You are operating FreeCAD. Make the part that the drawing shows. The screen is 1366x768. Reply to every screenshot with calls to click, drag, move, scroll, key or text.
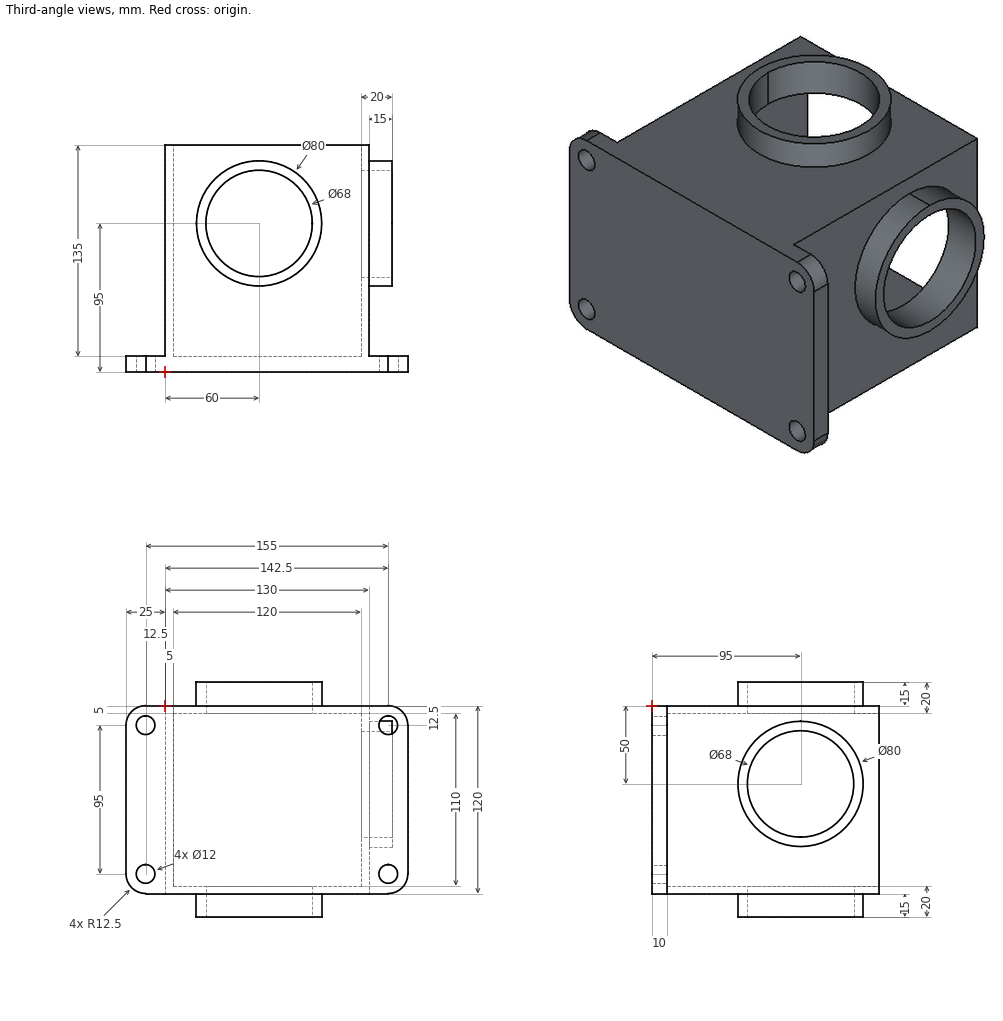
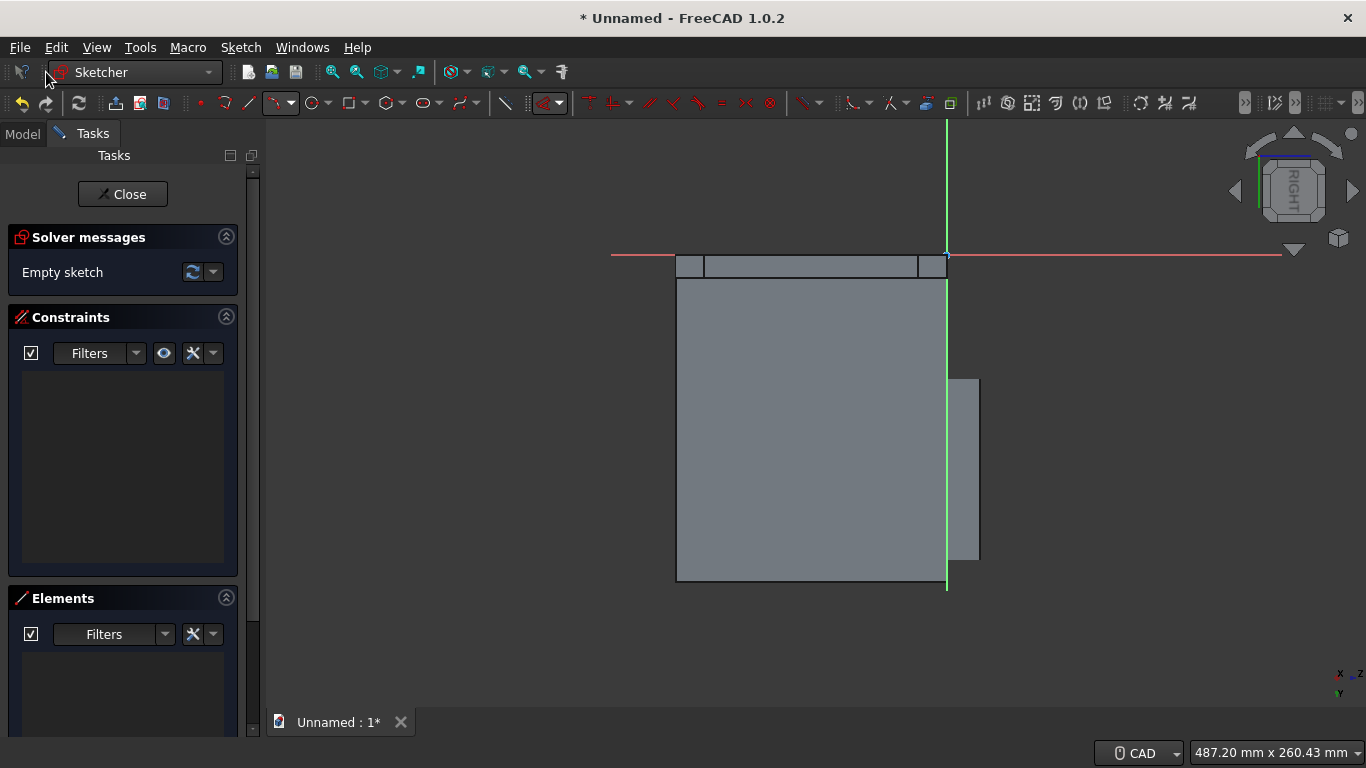
click(312, 104)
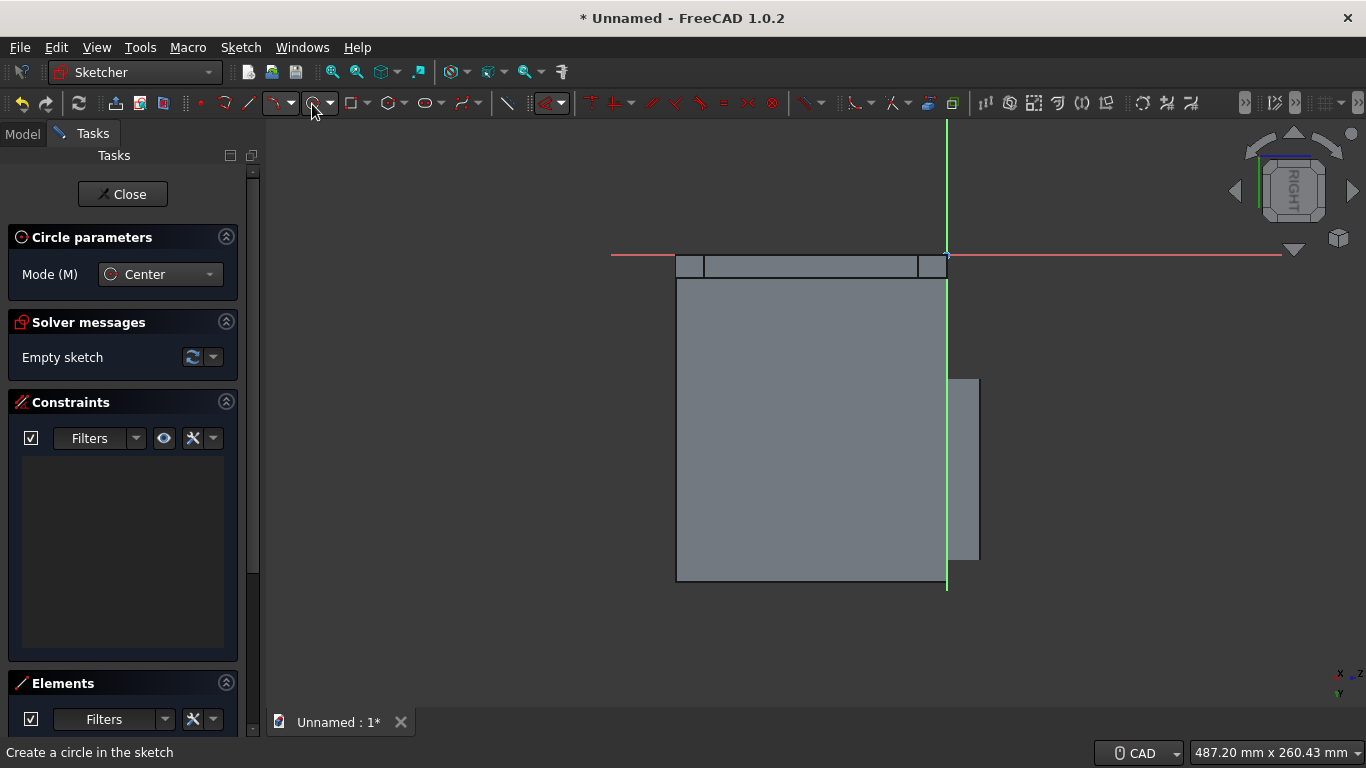
click(834, 470)
move(898, 406)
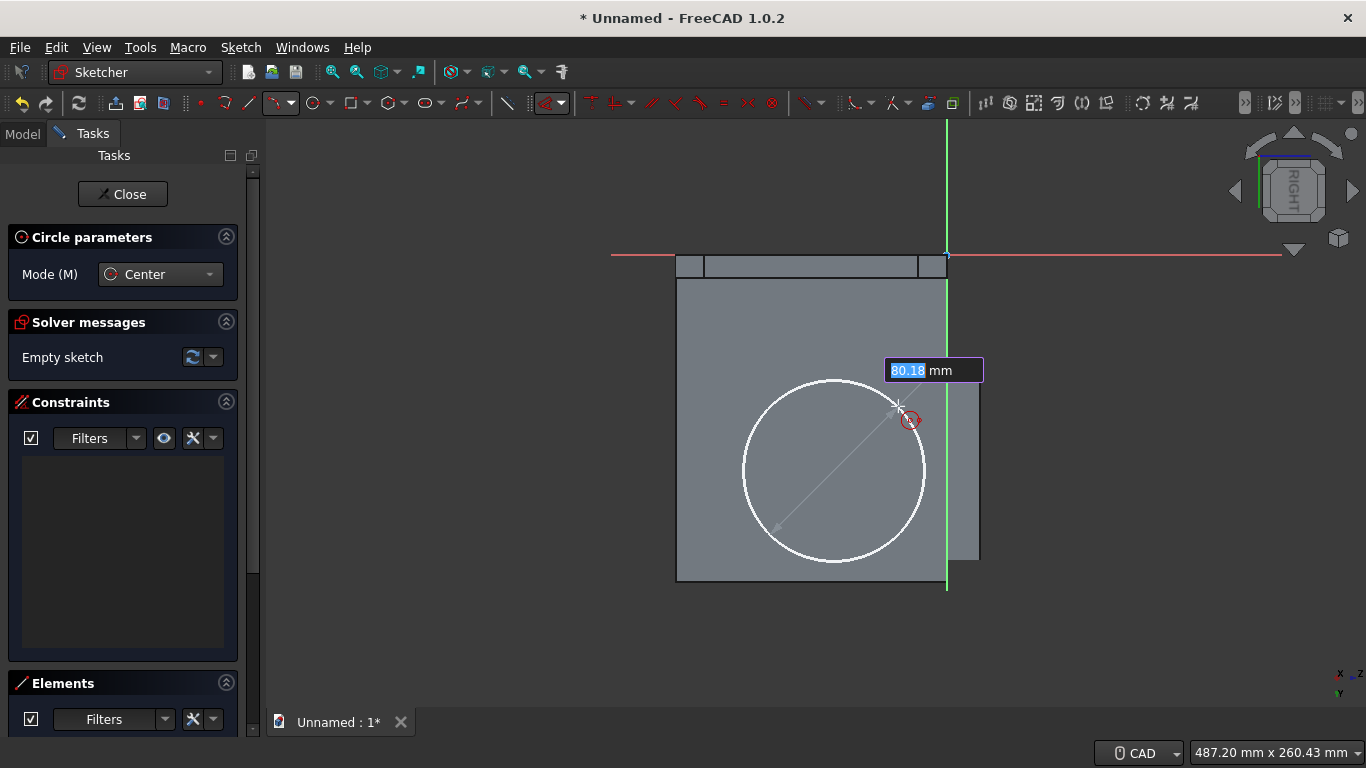
text(80)
key(Return)
key(Escape)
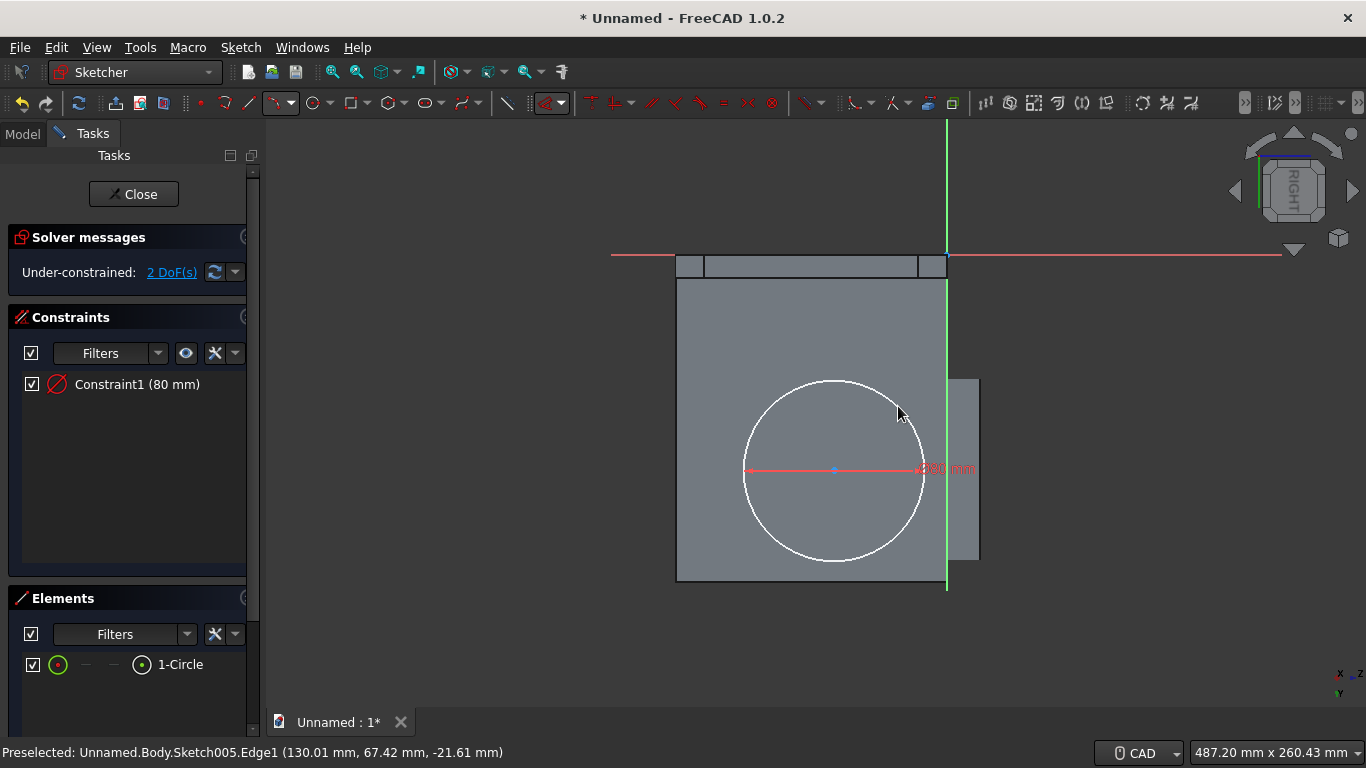
click(834, 471)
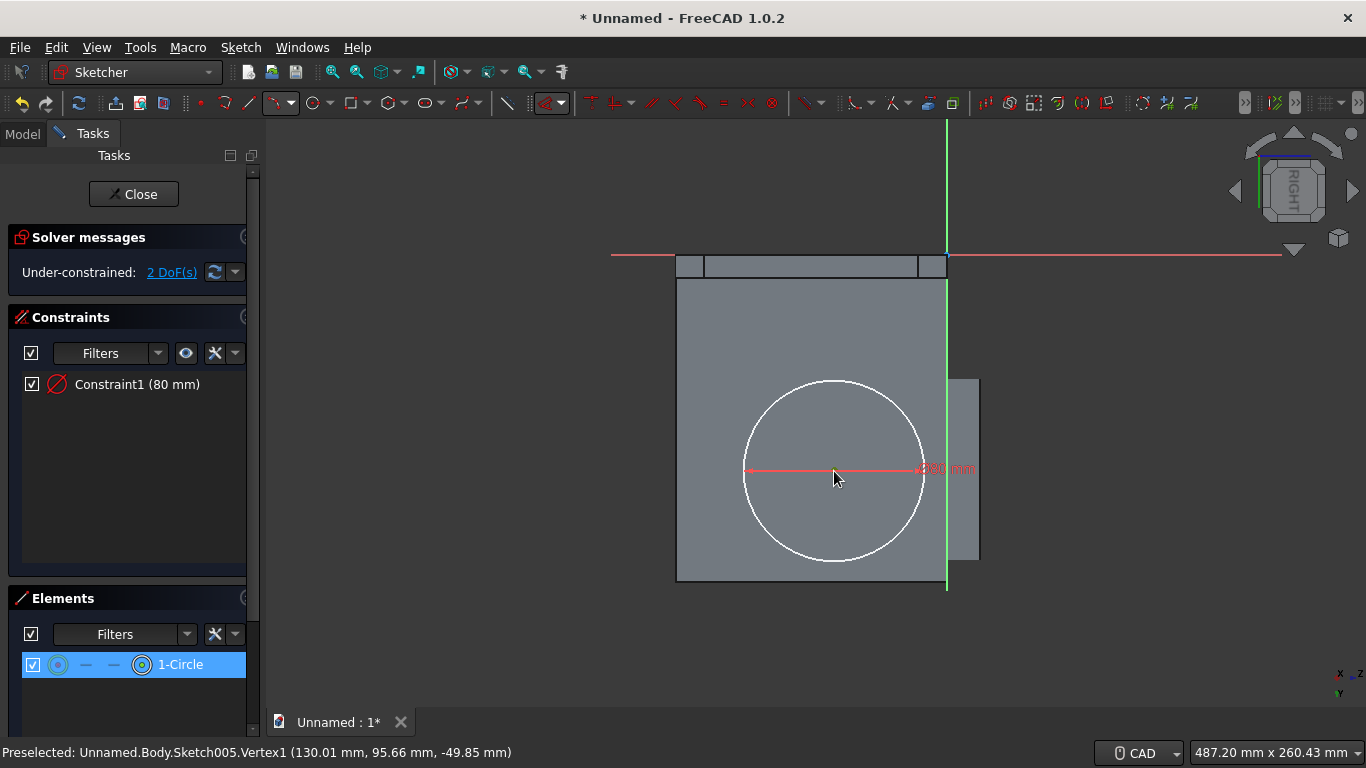
click(564, 104)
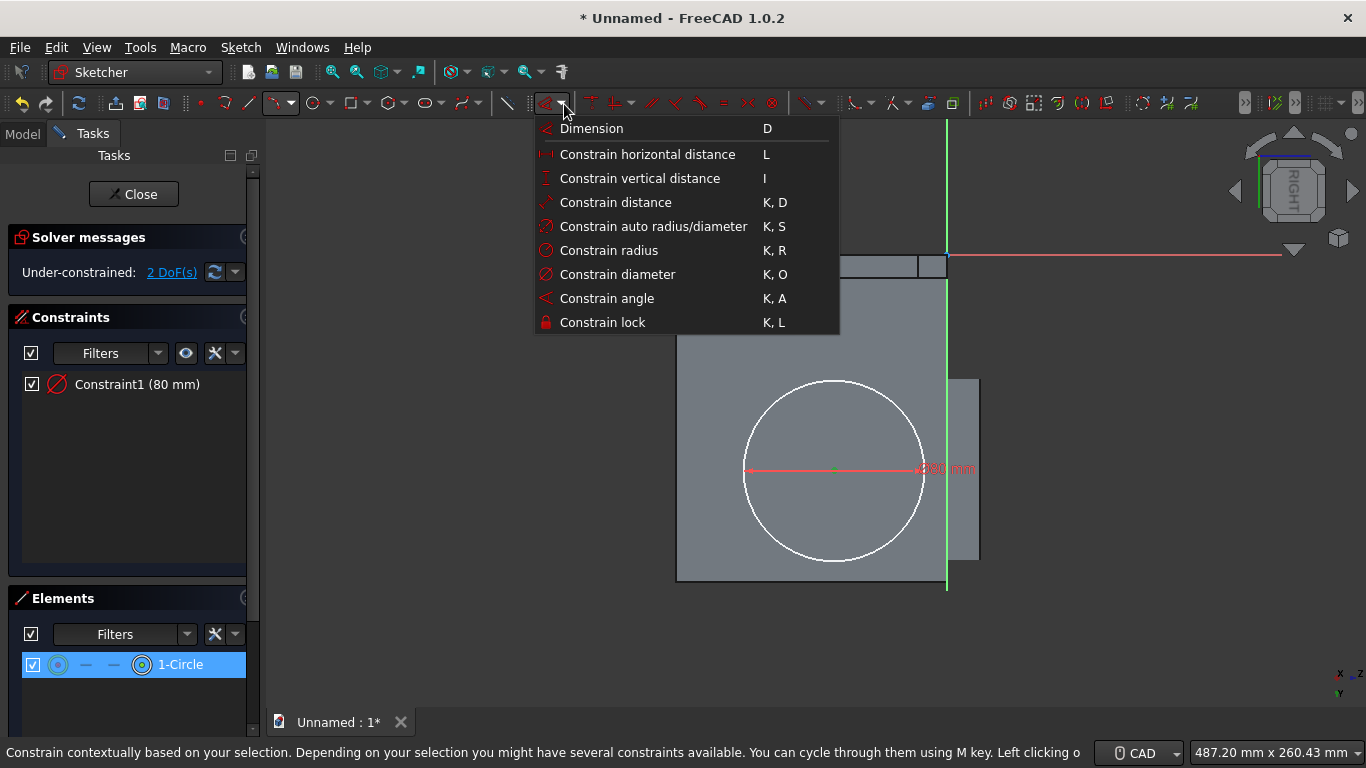
click(687, 154)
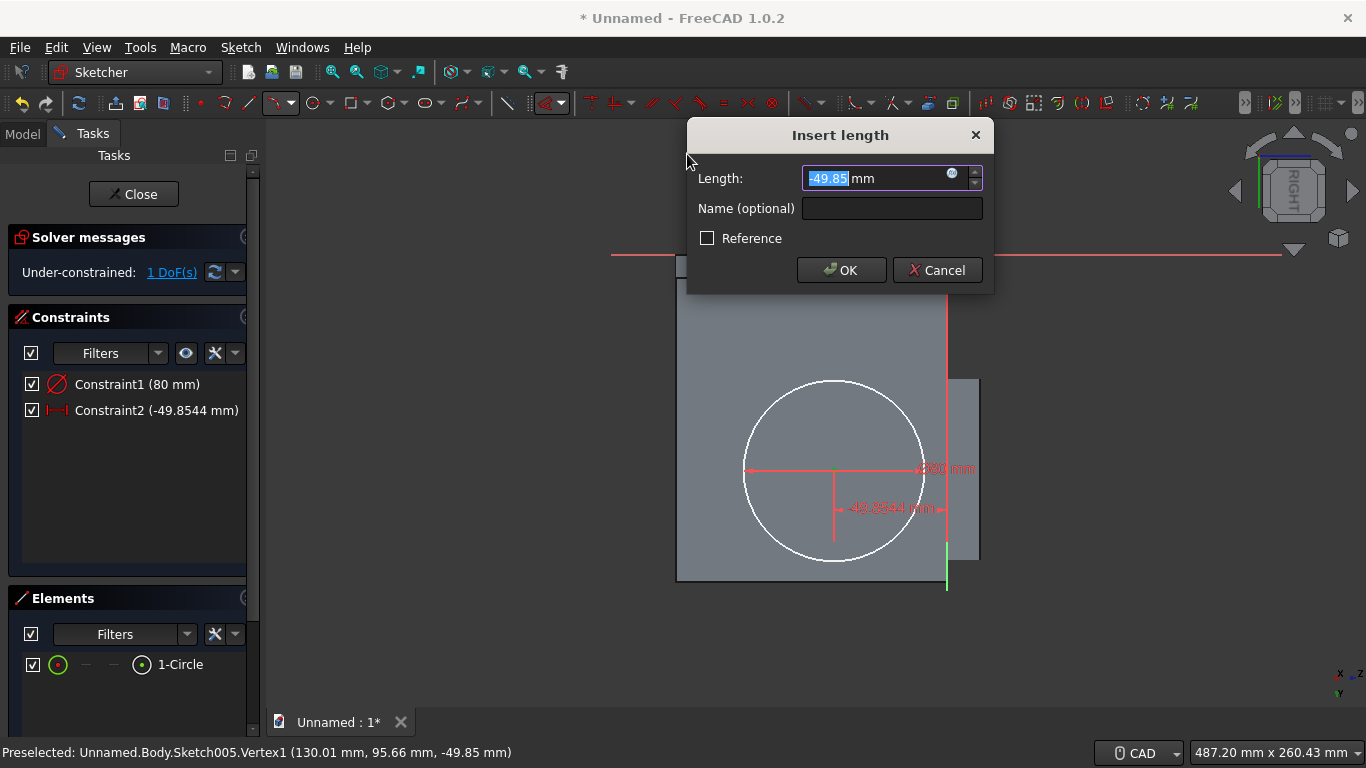
text(-50)
key(Return)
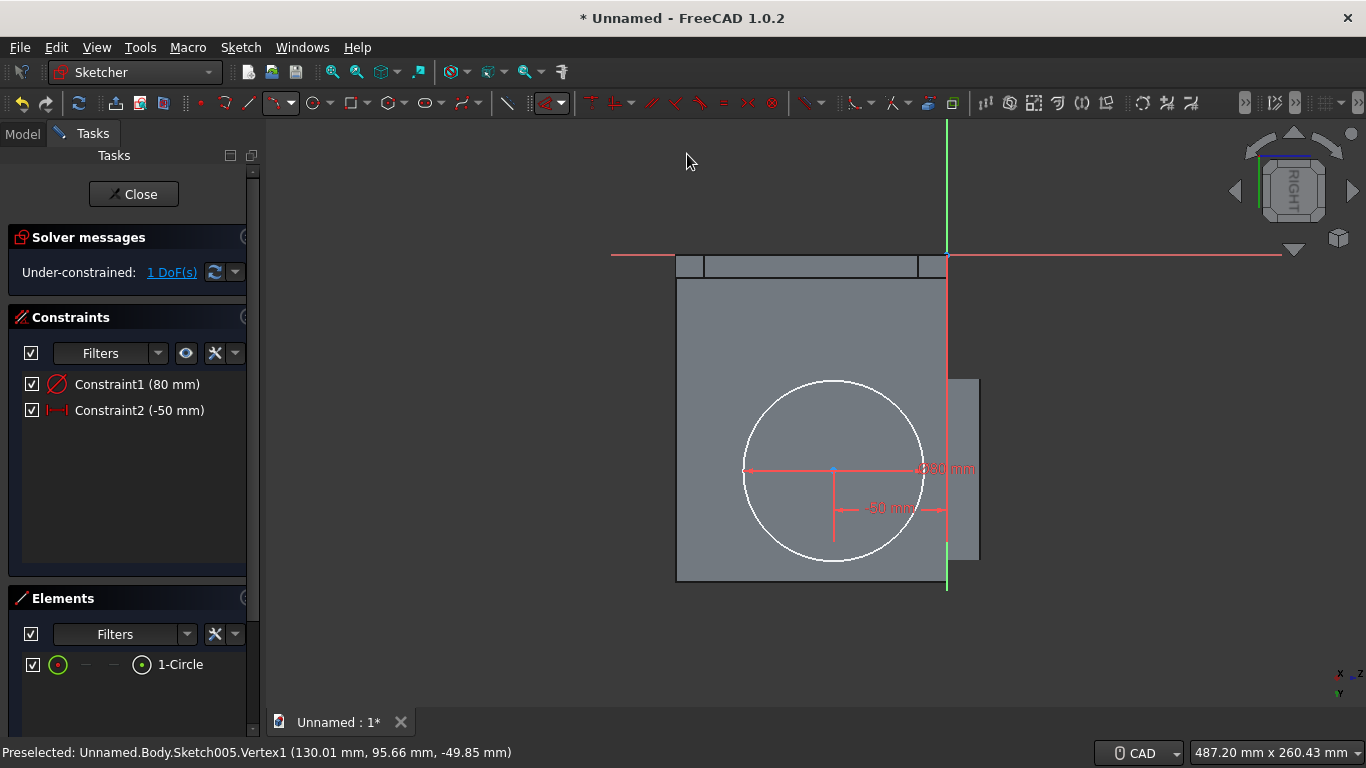
click(834, 471)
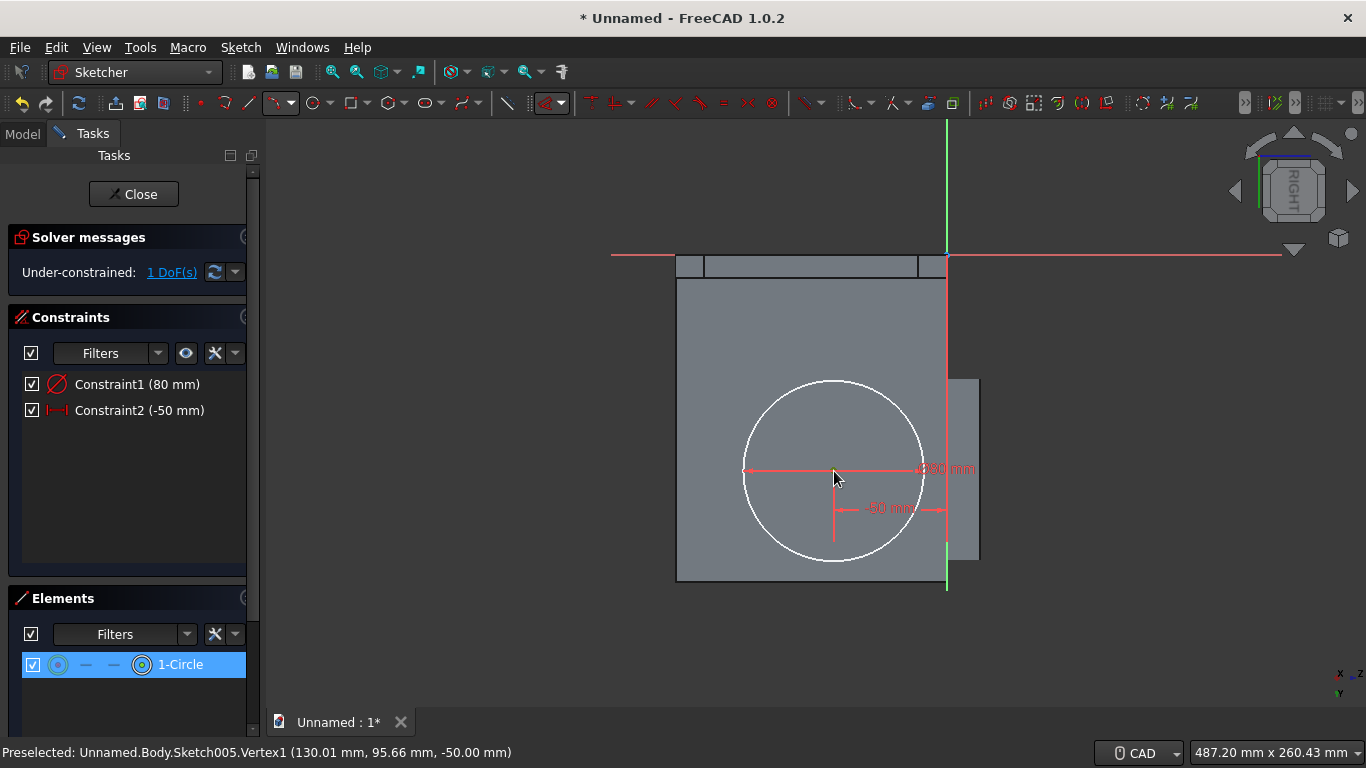
click(564, 104)